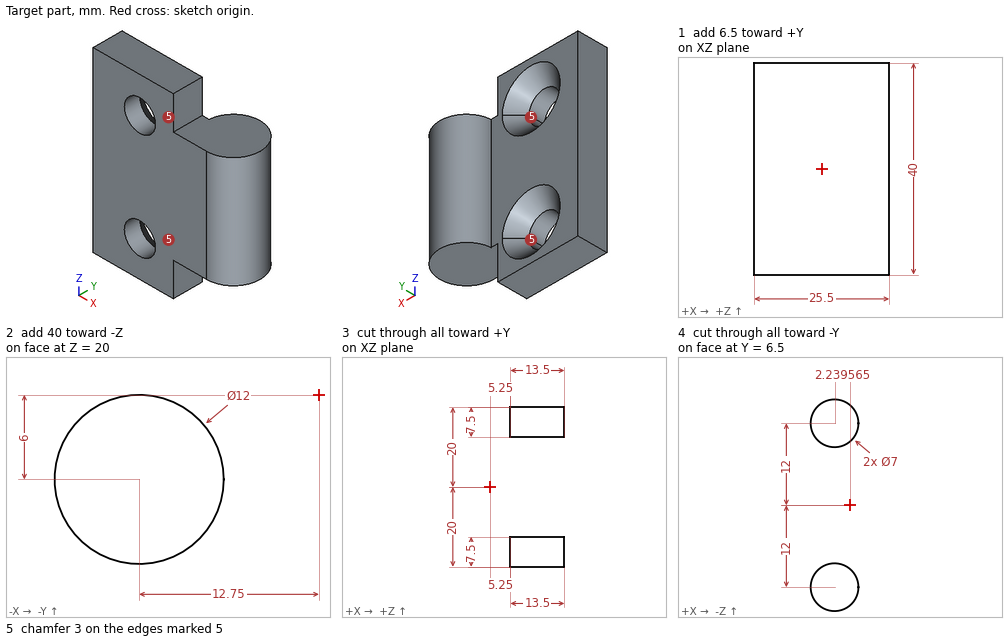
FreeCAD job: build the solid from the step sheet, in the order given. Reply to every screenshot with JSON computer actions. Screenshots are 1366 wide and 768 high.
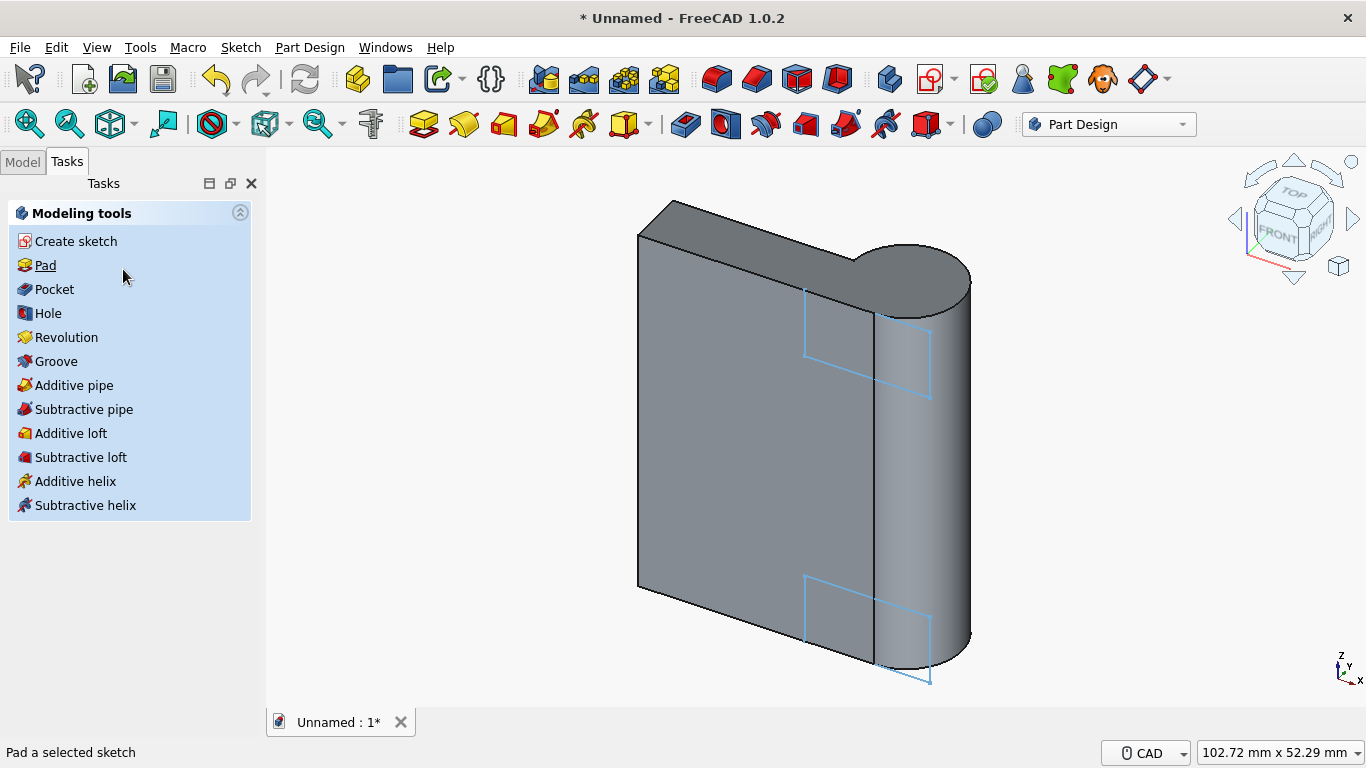
{"action": "left_click", "coordinate": [686, 124]}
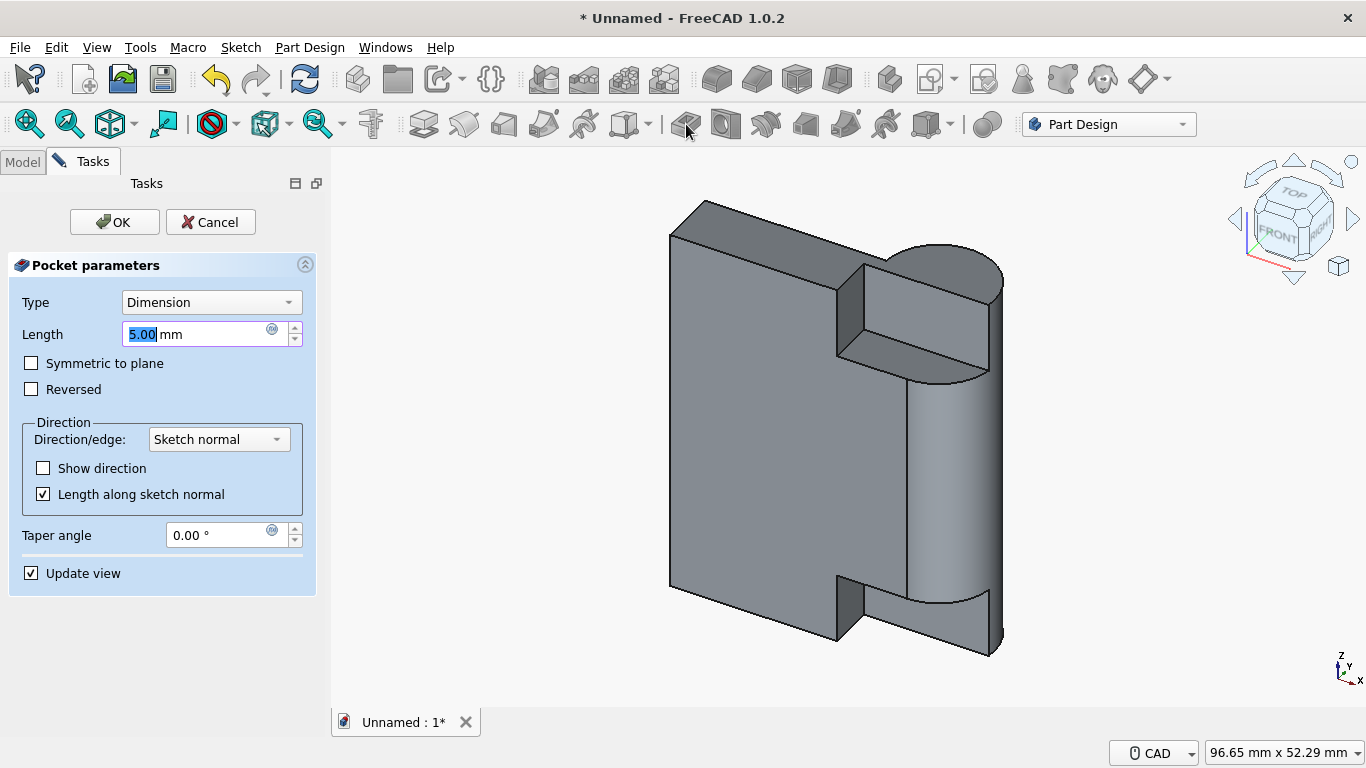
{"action": "left_click", "coordinate": [212, 302]}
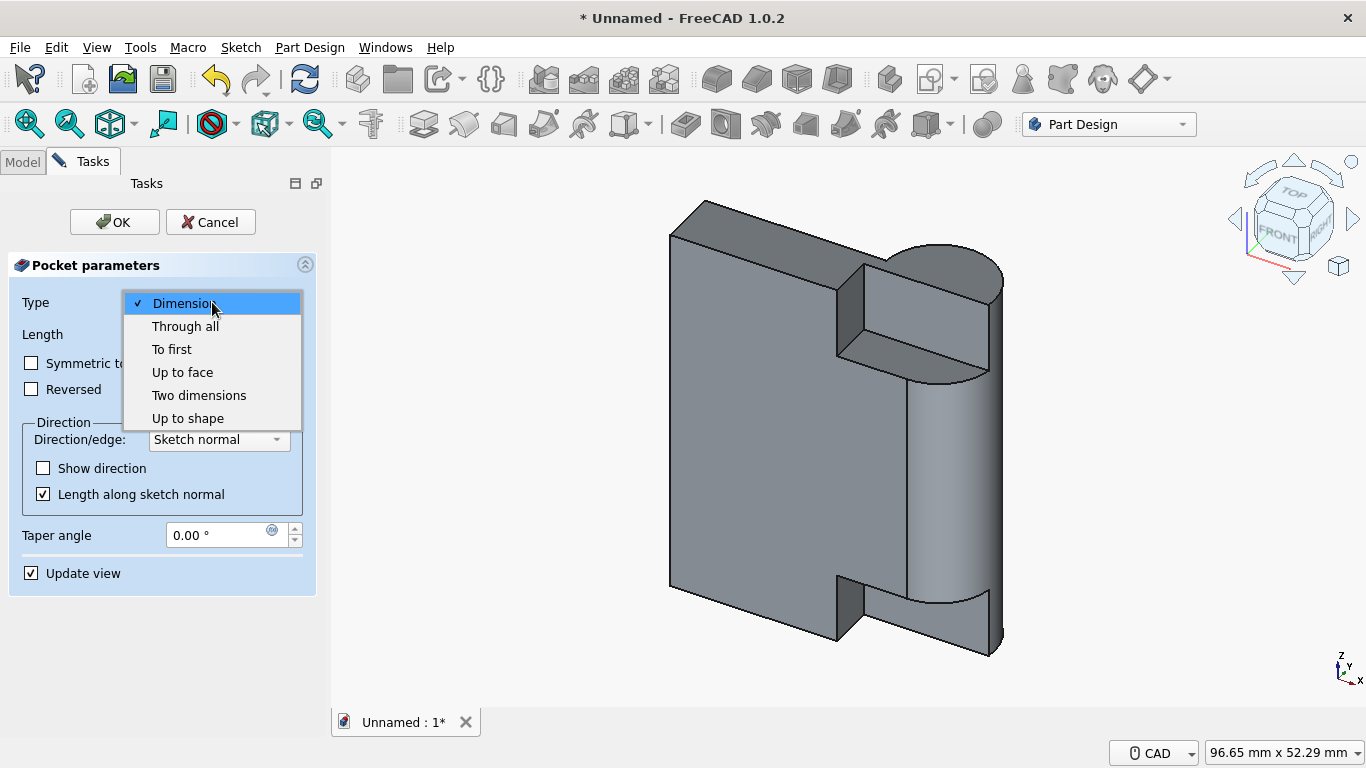
{"action": "left_click", "coordinate": [212, 326]}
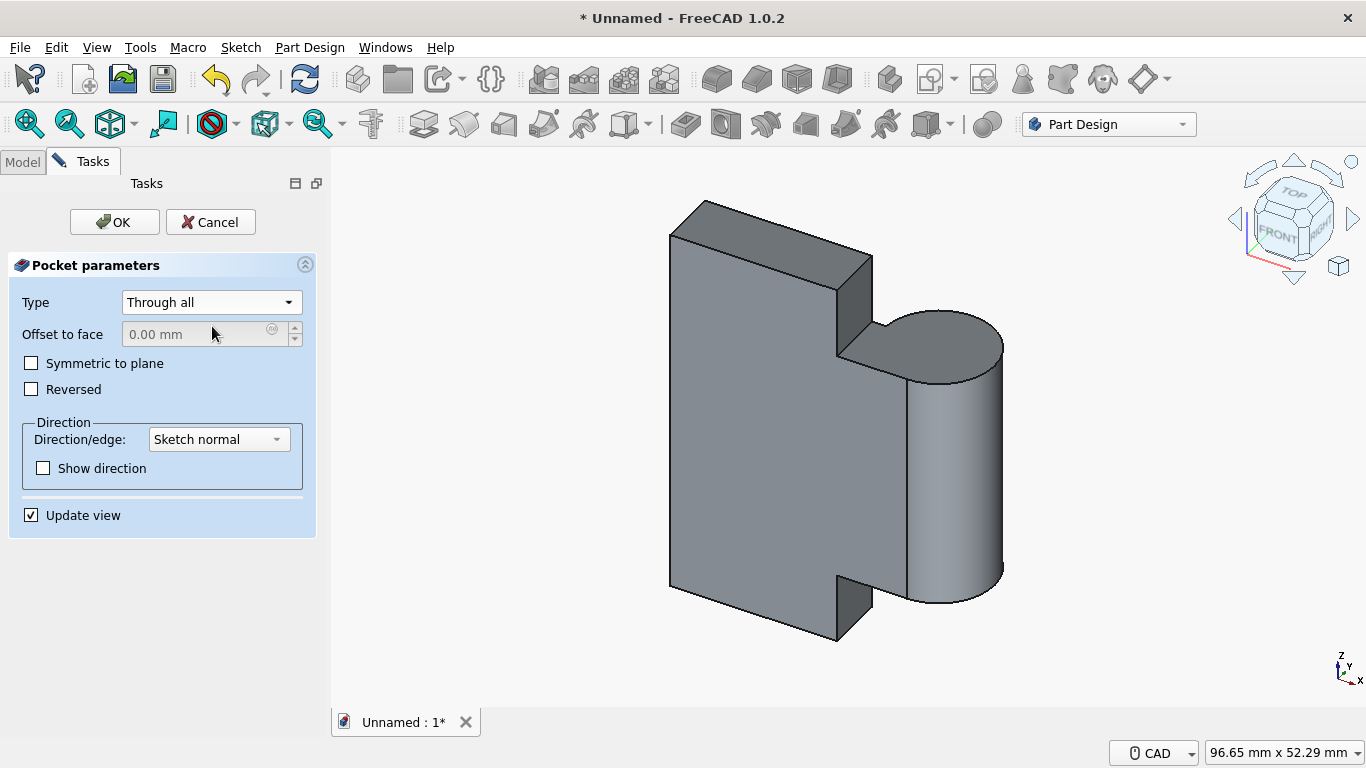
{"action": "left_click", "coordinate": [115, 222]}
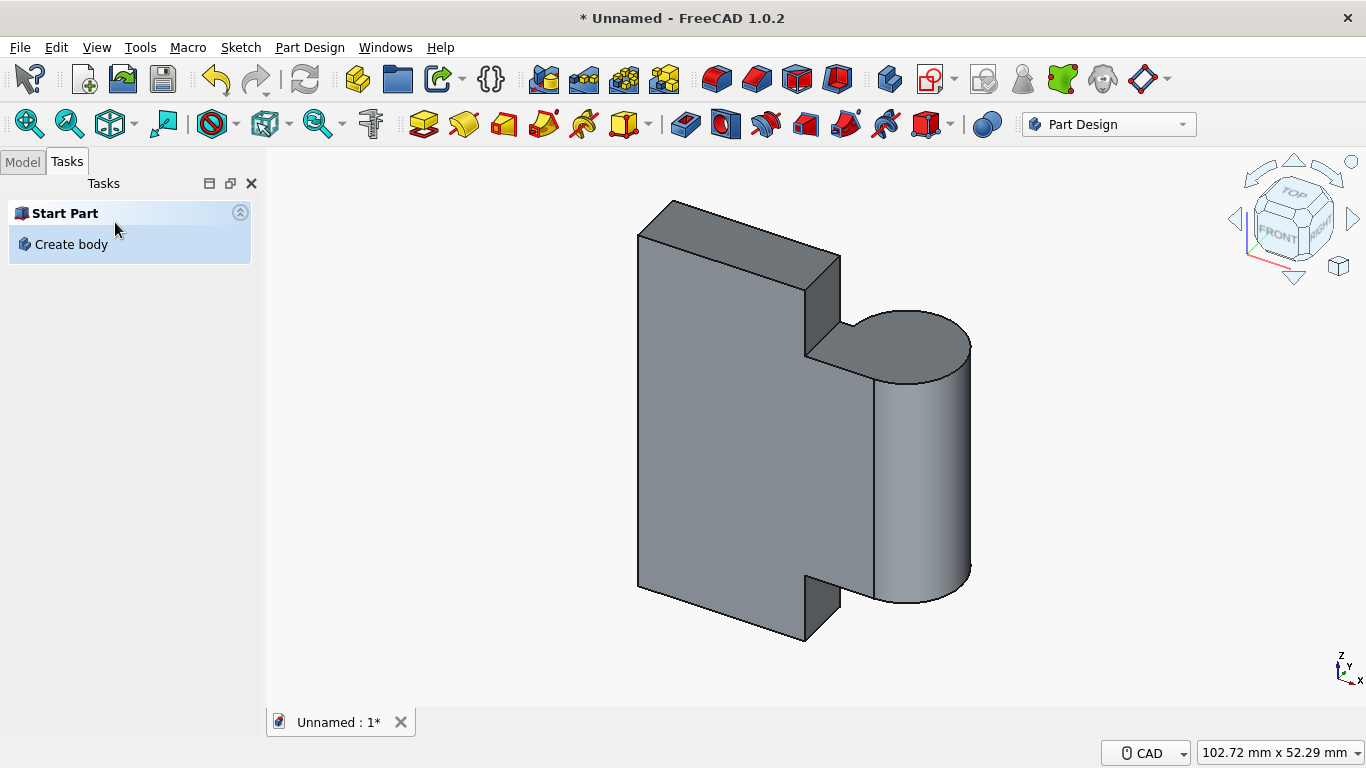
{"action": "key", "text": "4"}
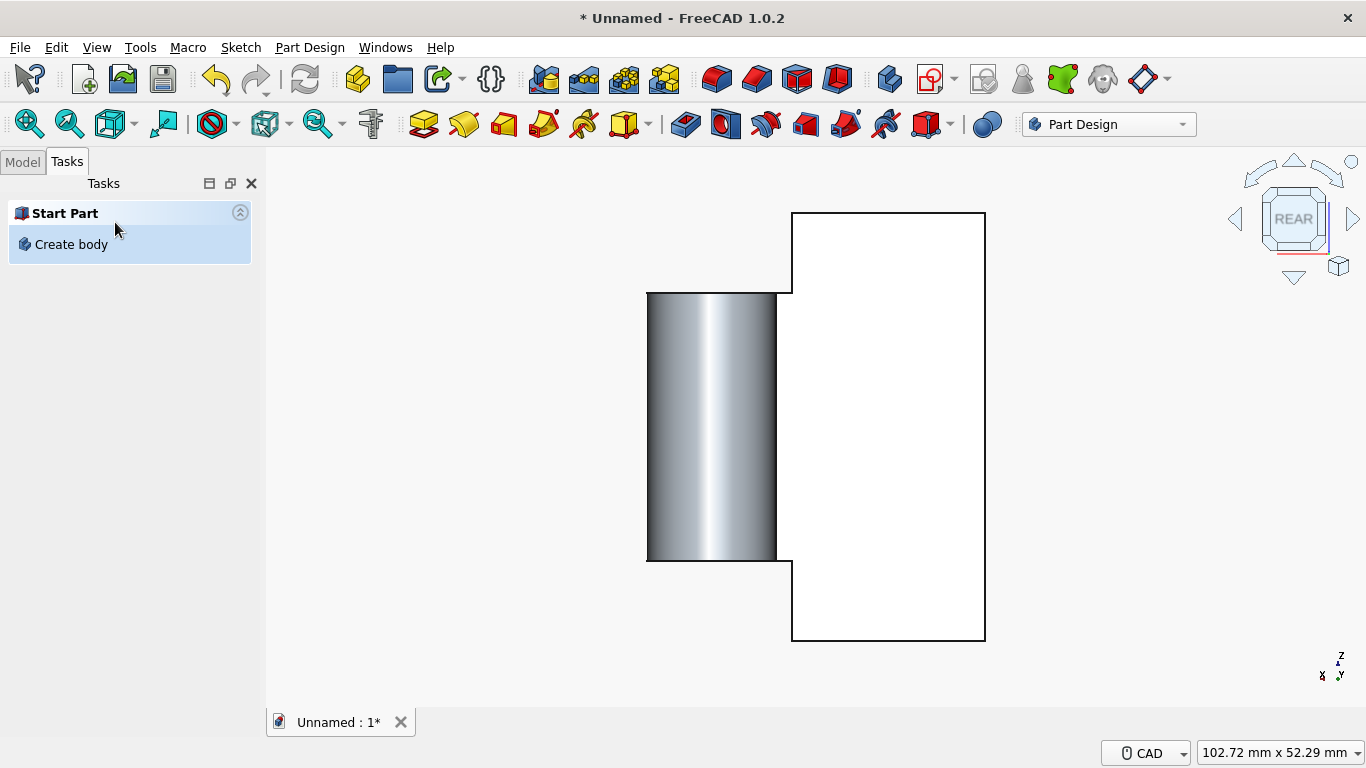
{"action": "left_click", "coordinate": [880, 365]}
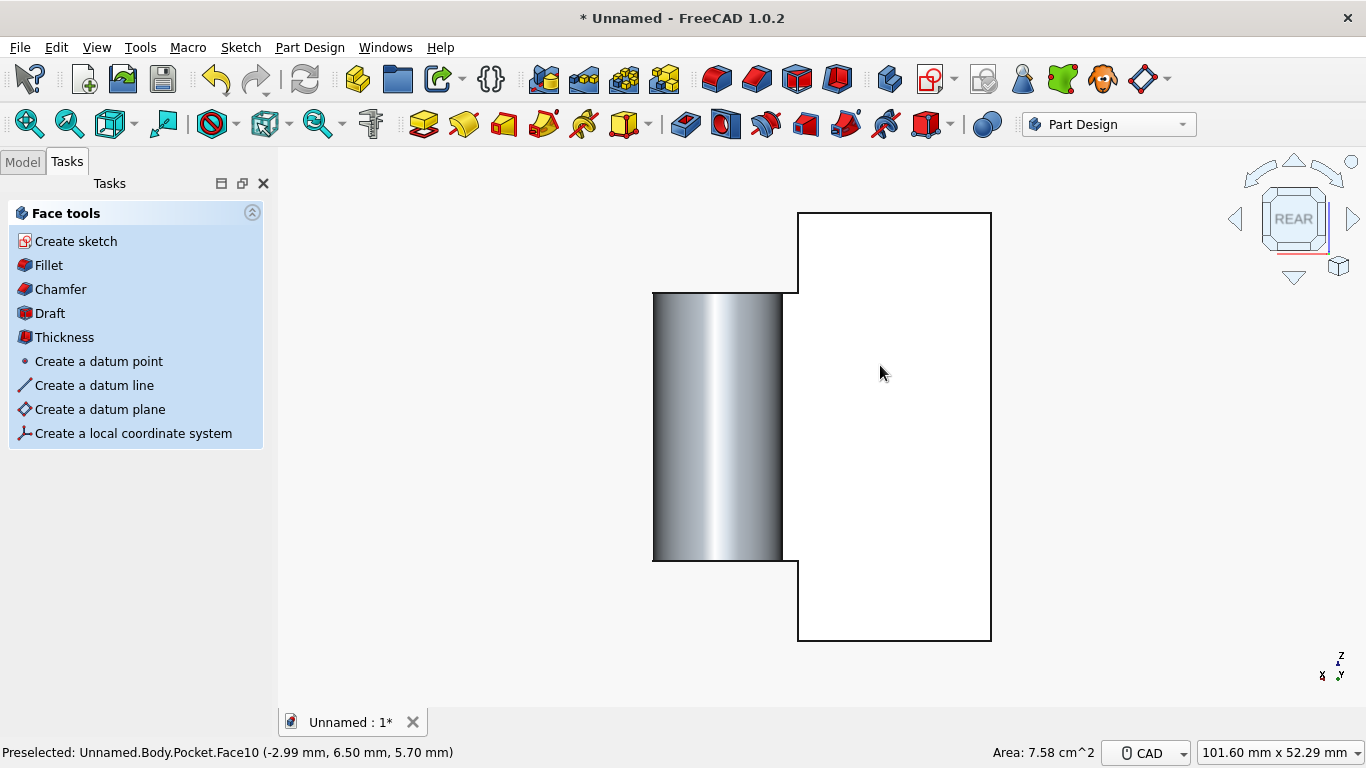
{"action": "left_click", "coordinate": [930, 80]}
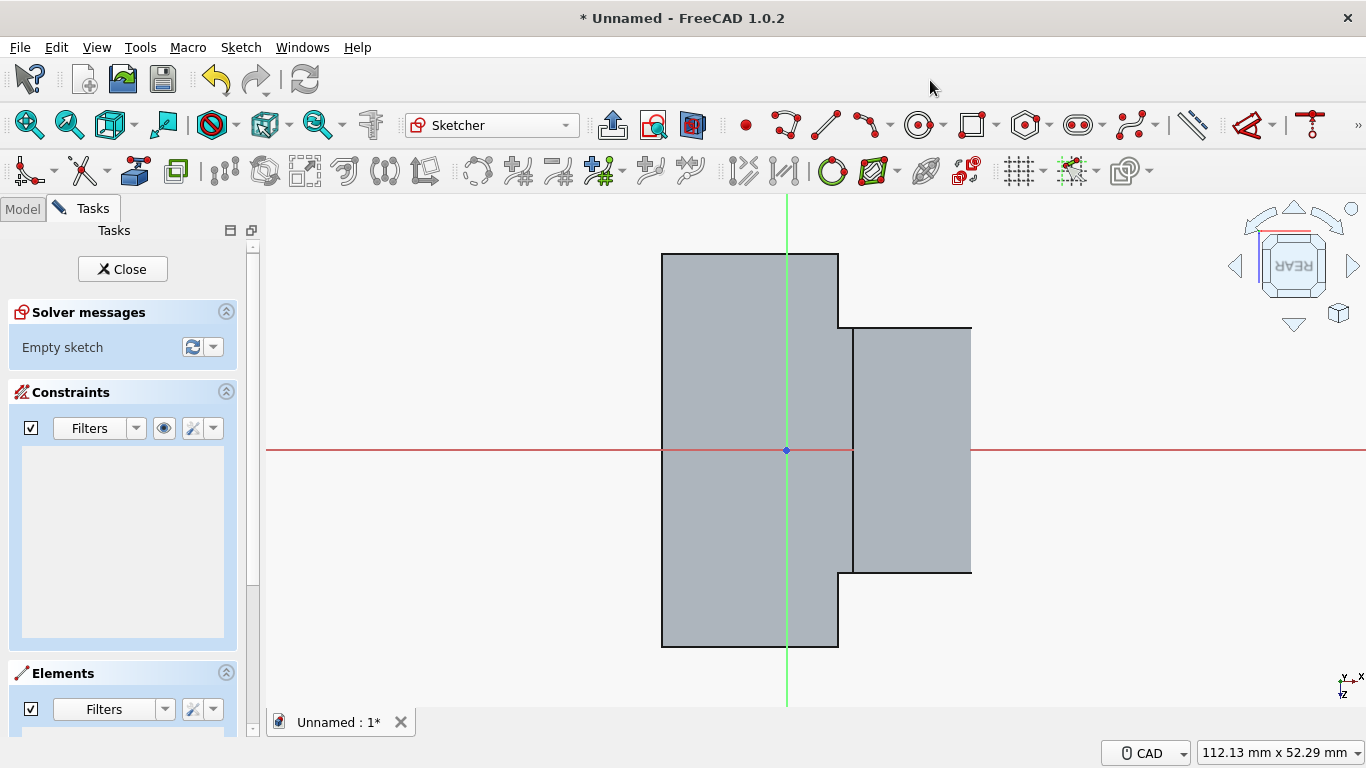
{"action": "left_click", "coordinate": [694, 126]}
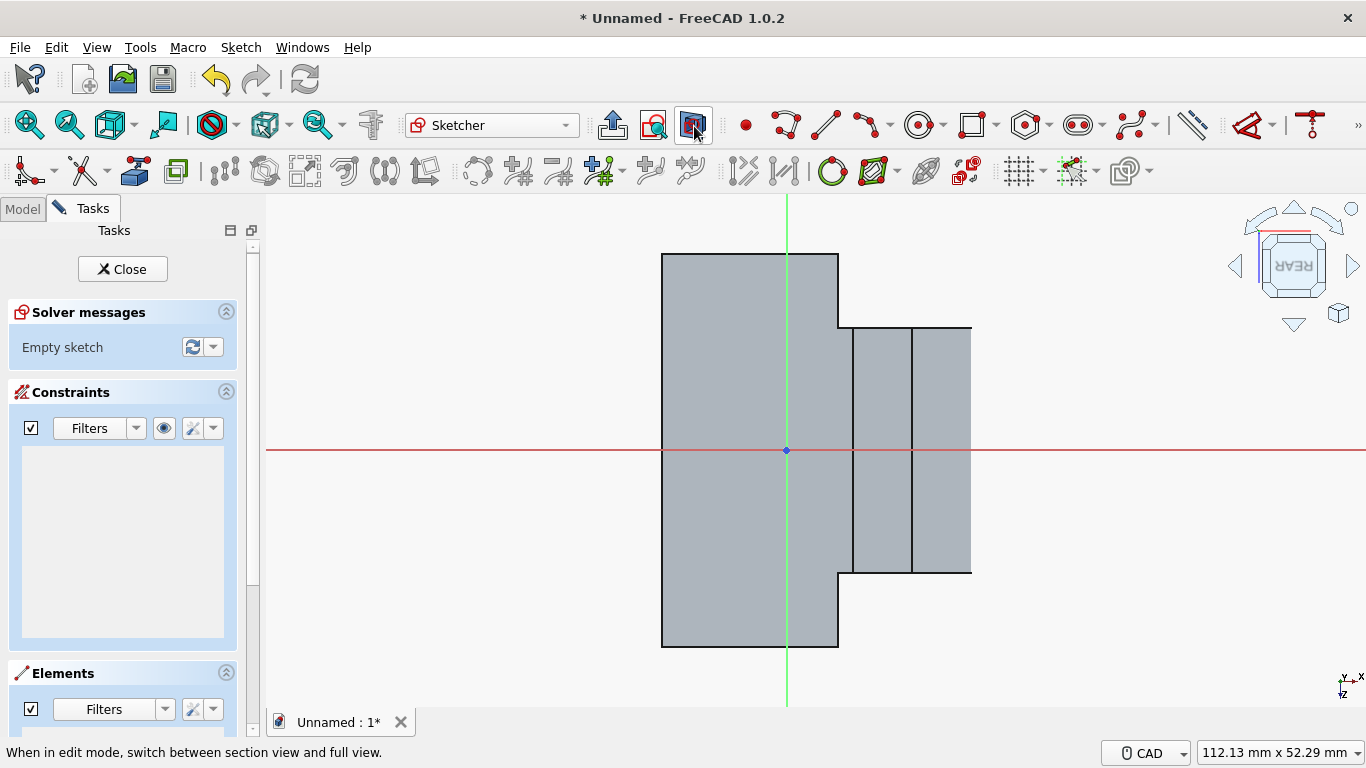
{"action": "left_click", "coordinate": [920, 126]}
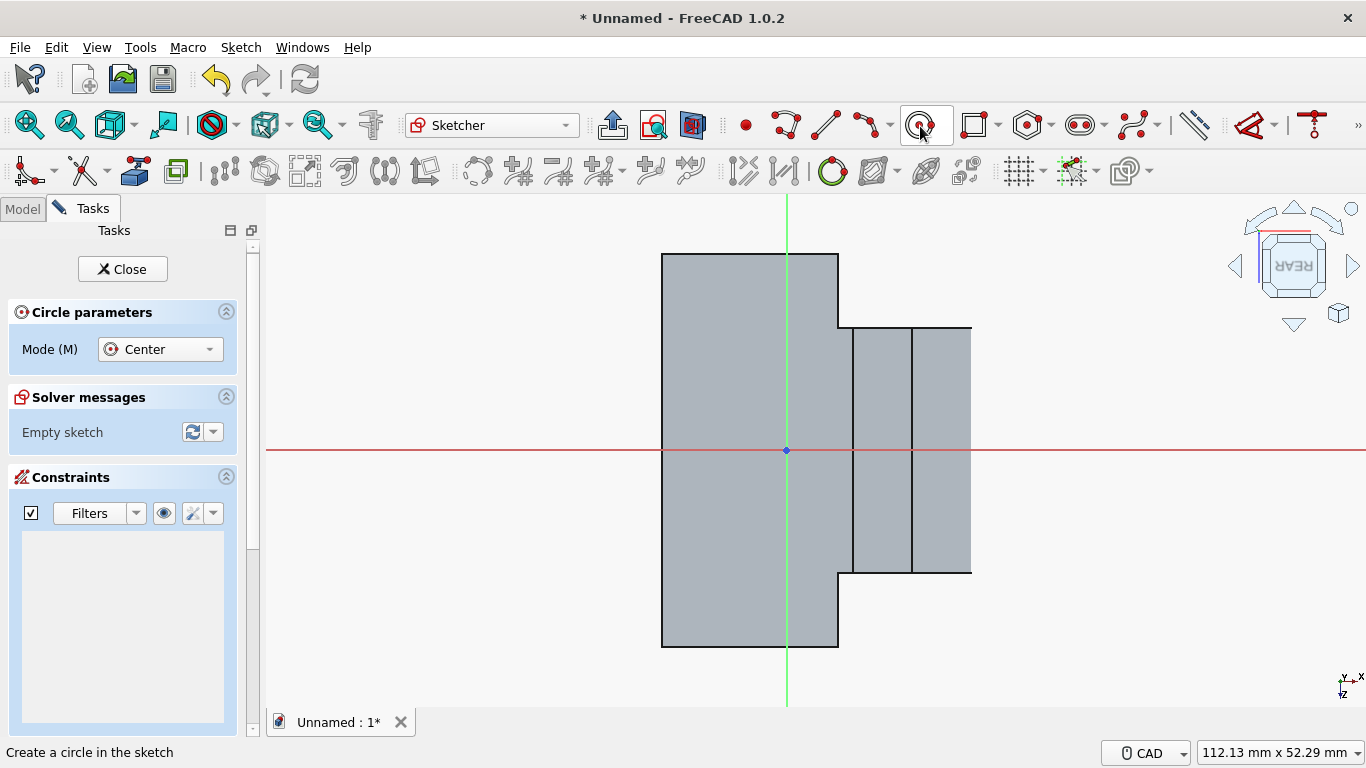
{"action": "left_click", "coordinate": [765, 333]}
{"action": "left_click", "coordinate": [740, 308]}